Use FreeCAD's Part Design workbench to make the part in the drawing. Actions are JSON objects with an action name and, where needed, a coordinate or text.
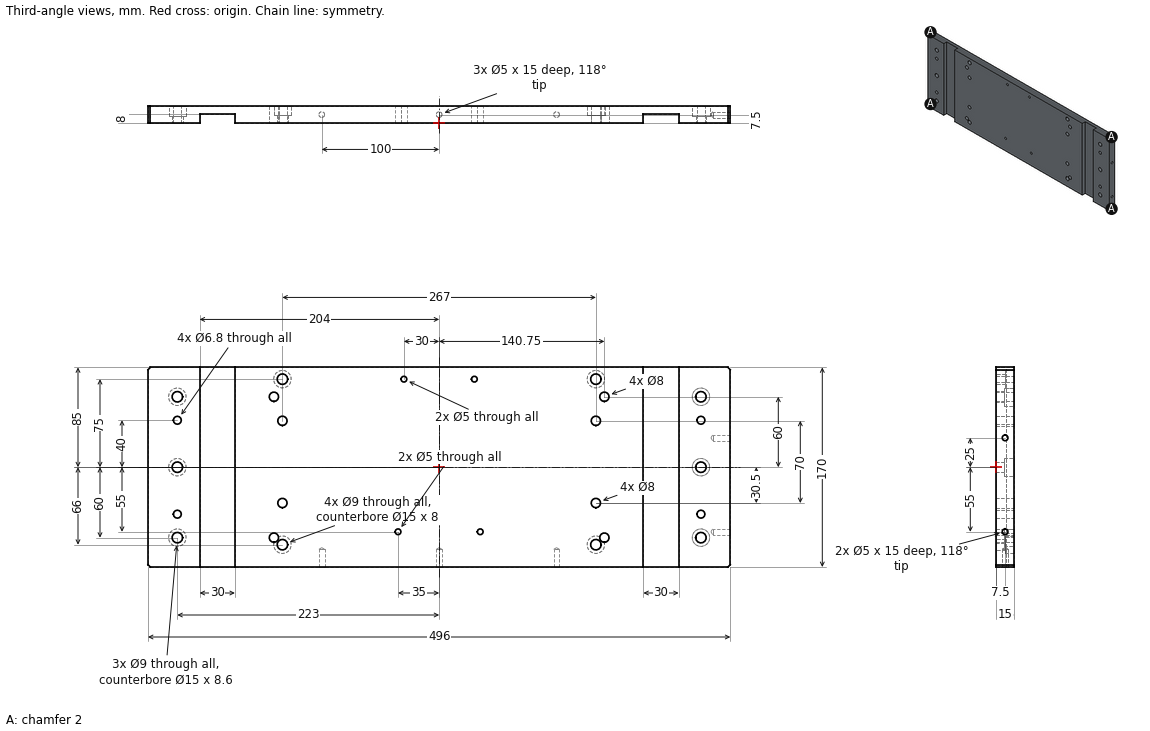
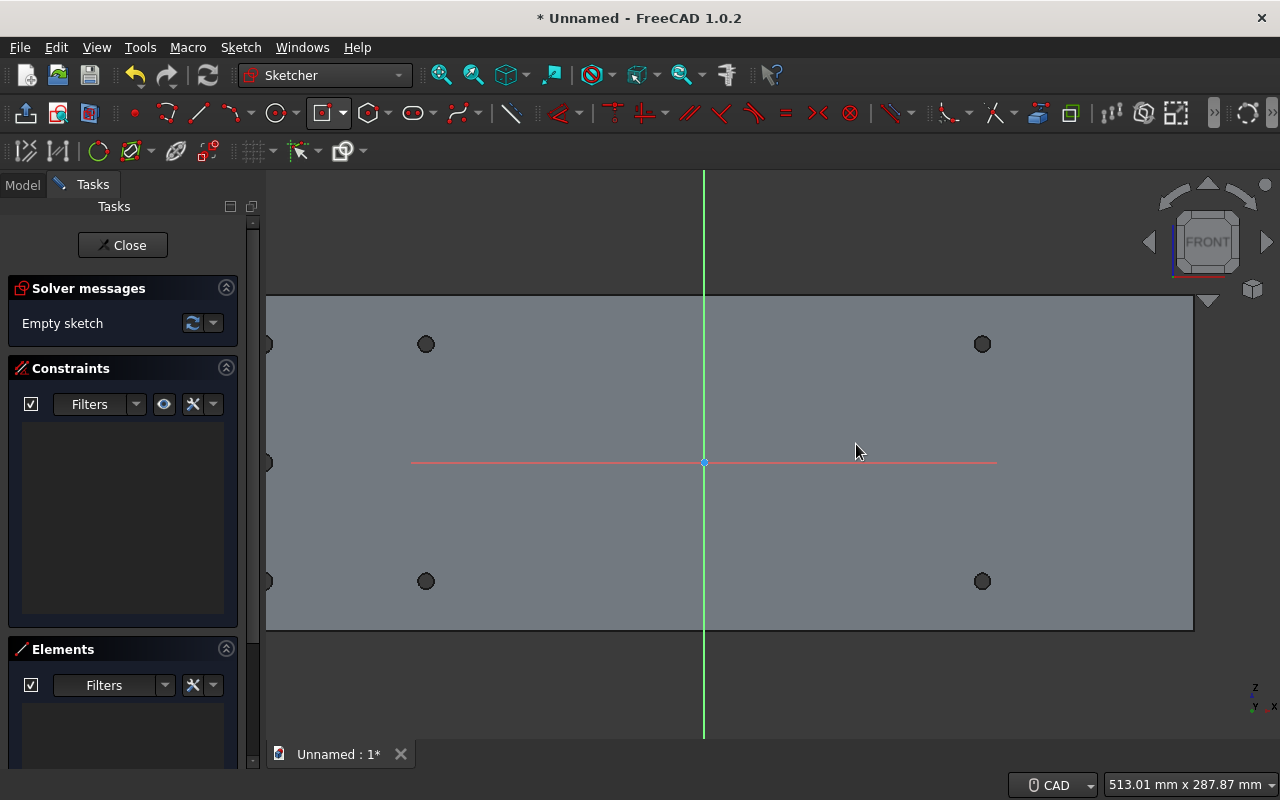
{"action": "left_click", "coordinate": [276, 114]}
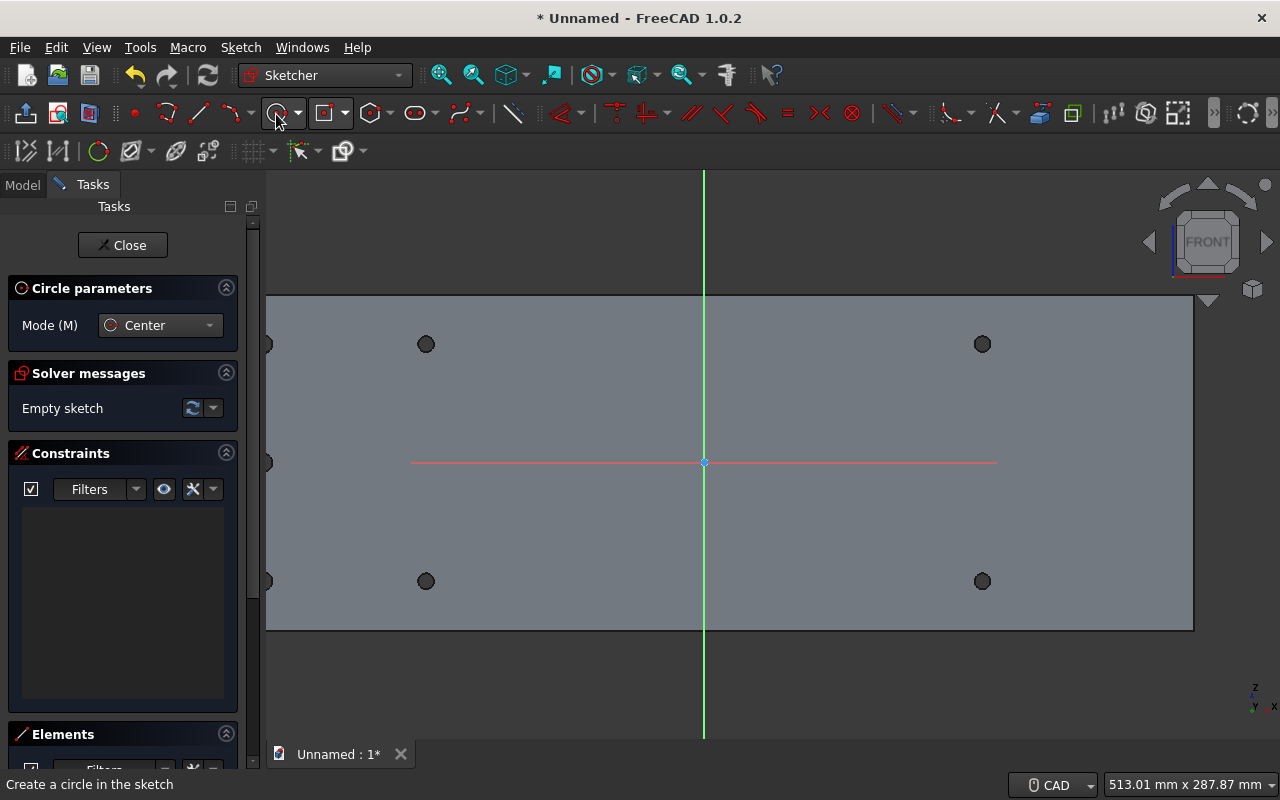
{"action": "scroll", "coordinate": [968, 523], "scroll_direction": "up", "scroll_amount": 6}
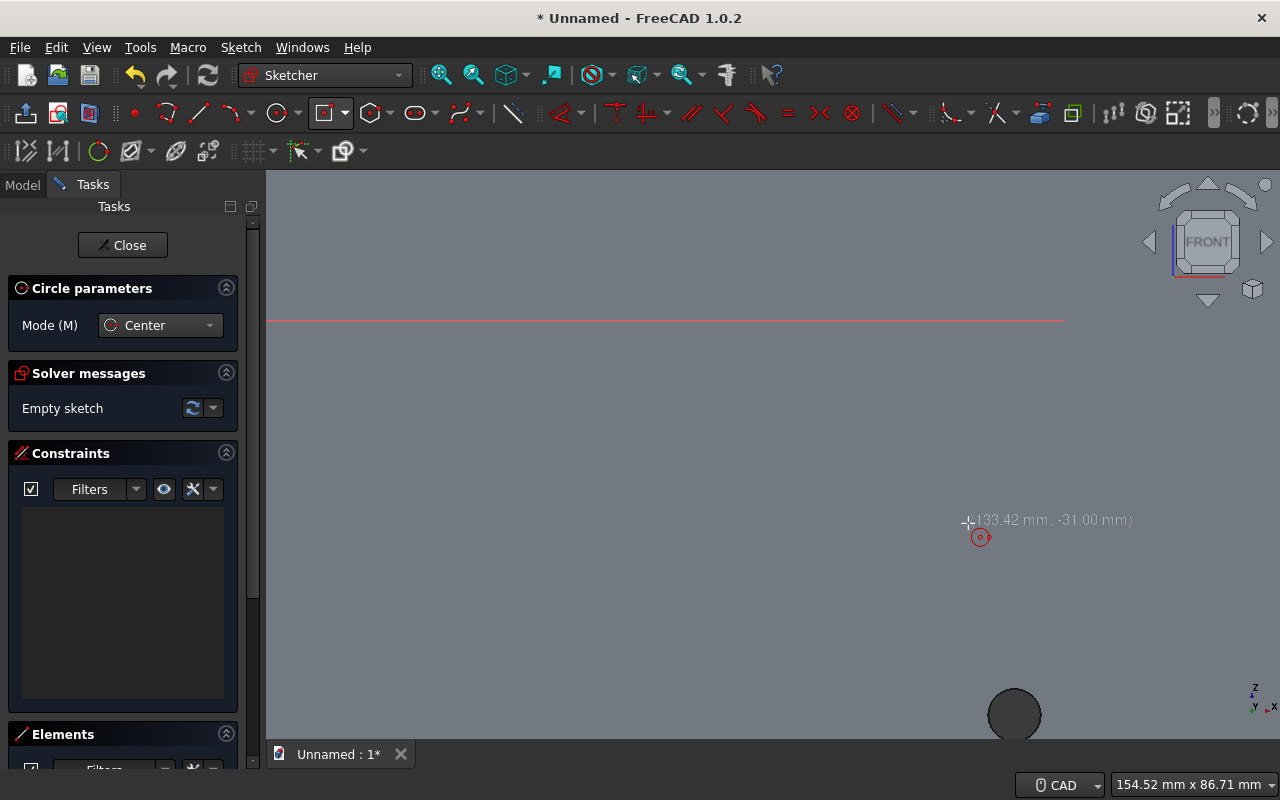
{"action": "left_click", "coordinate": [967, 522]}
{"action": "mouse_move", "coordinate": [985, 503]}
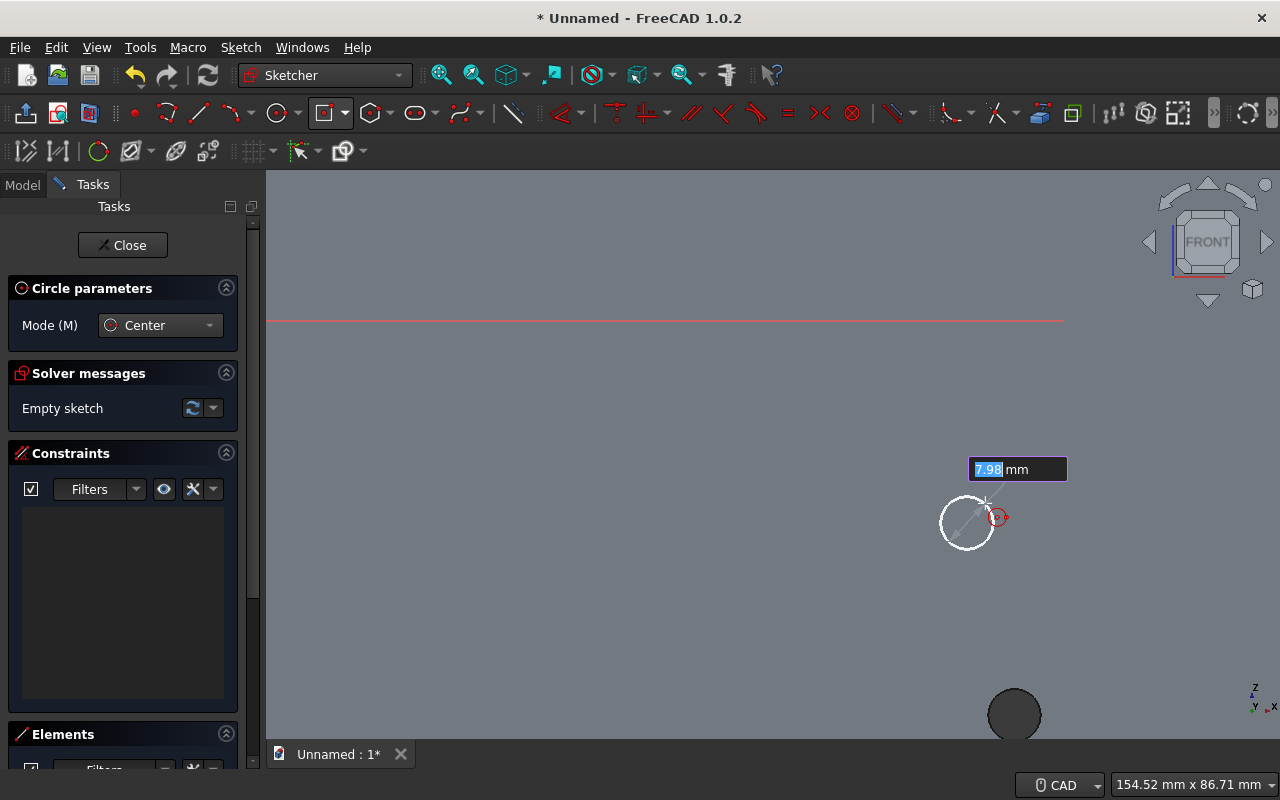
{"action": "type", "text": "8"}
{"action": "key", "text": "Return"}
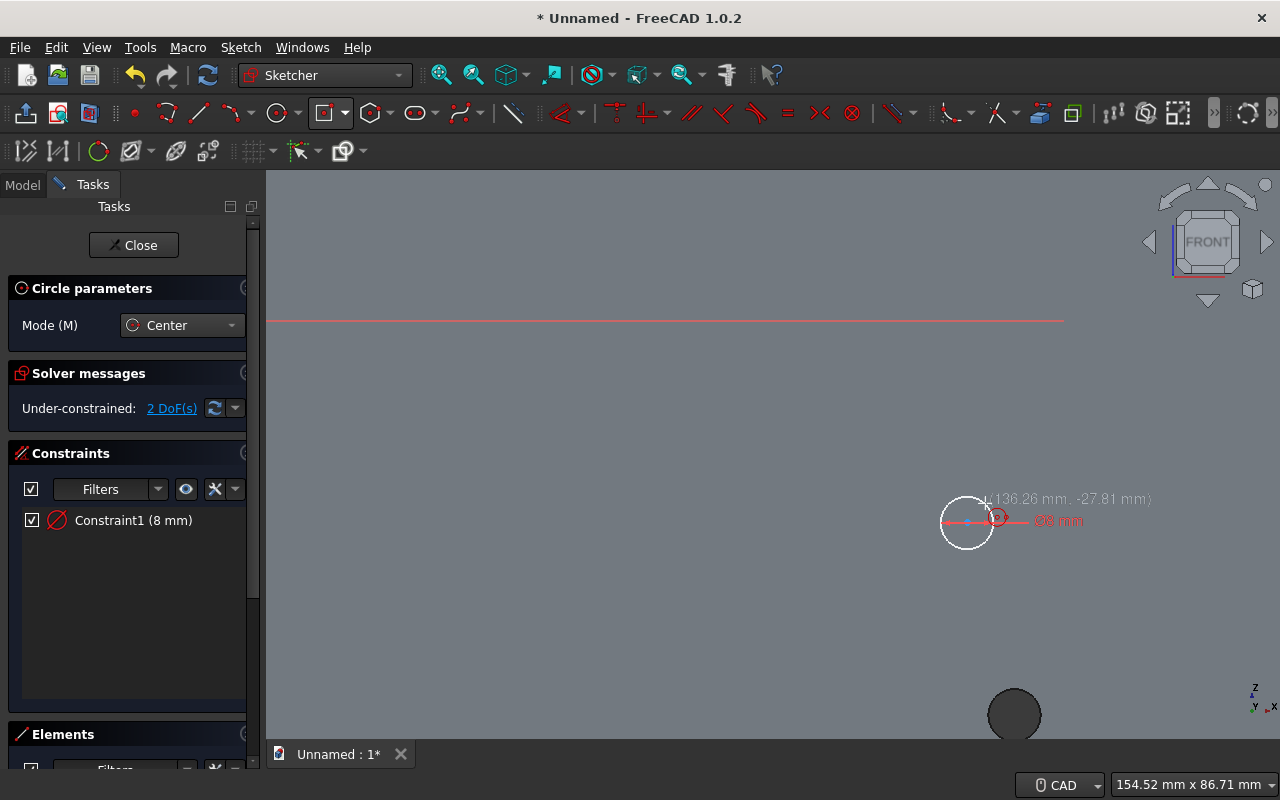
{"action": "scroll", "coordinate": [969, 525], "scroll_direction": "down", "scroll_amount": 6}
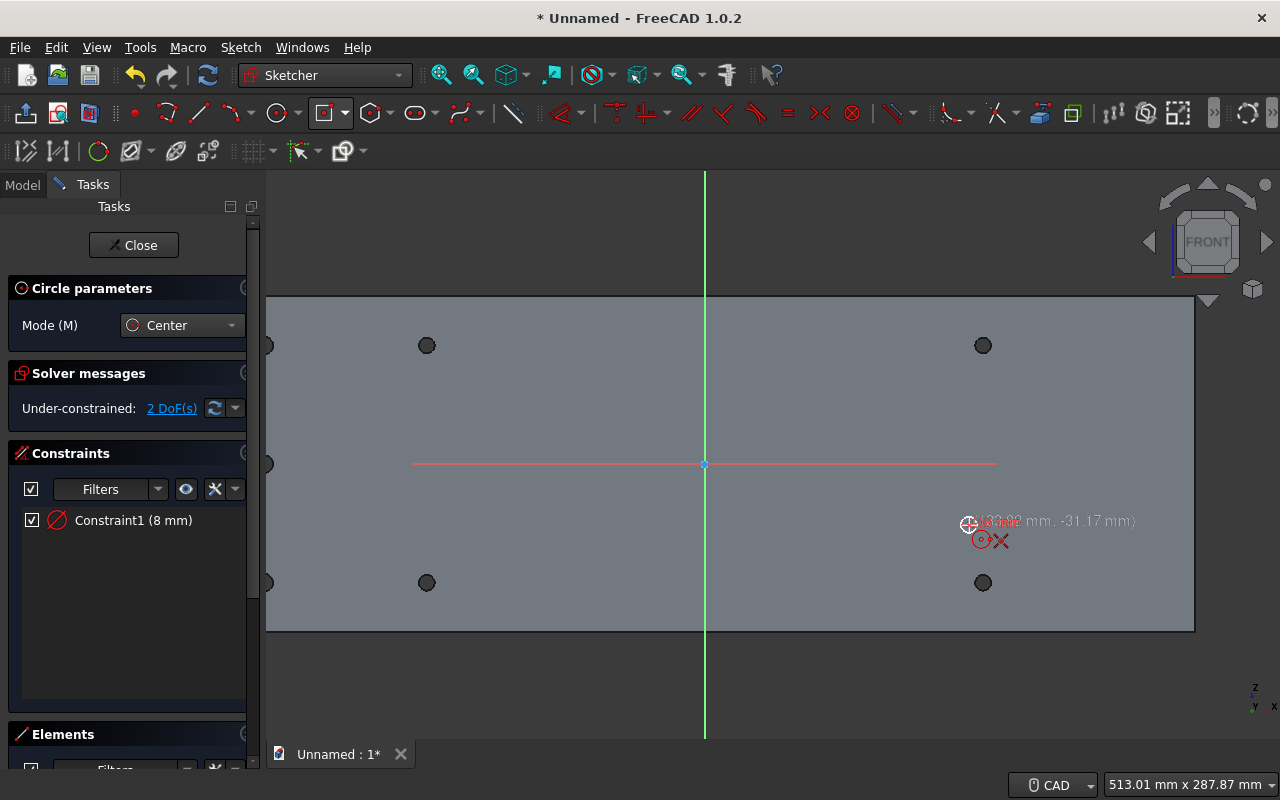
{"action": "scroll", "coordinate": [969, 386], "scroll_direction": "up", "scroll_amount": 6}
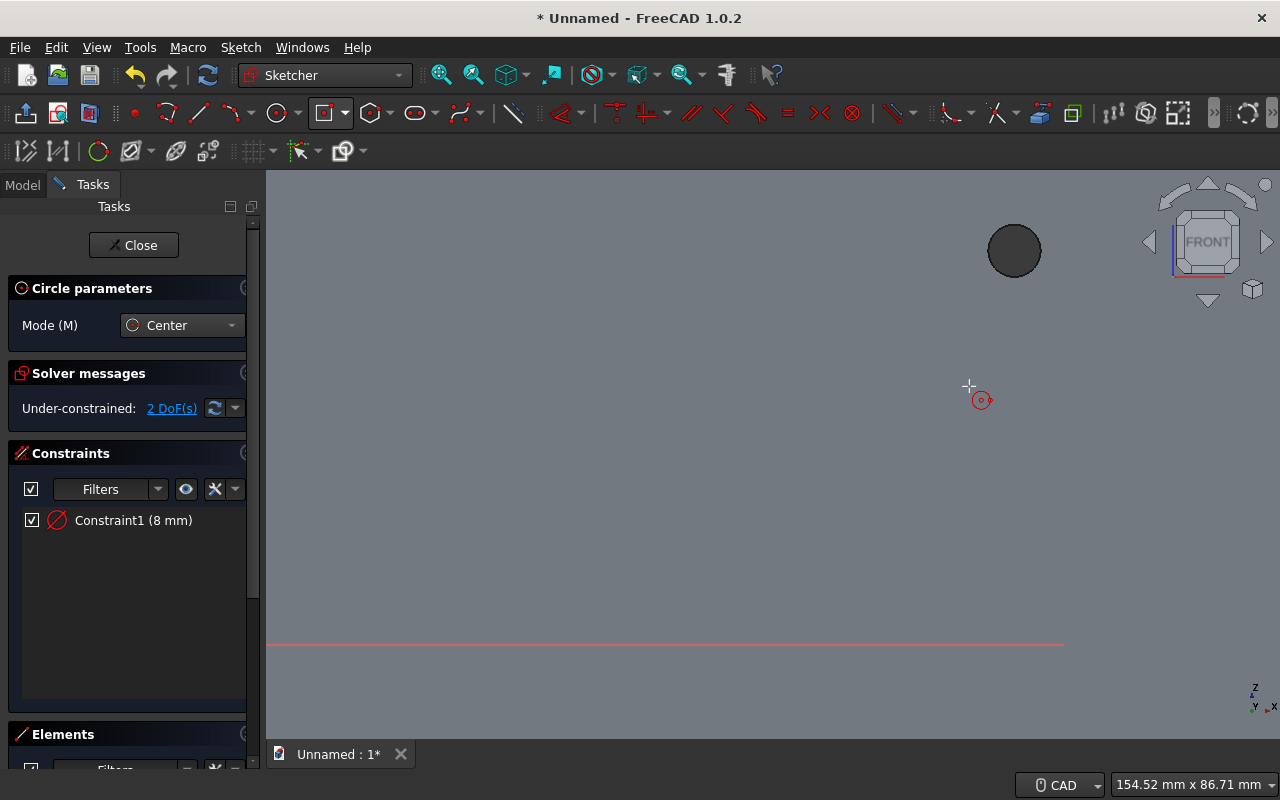
{"action": "left_click", "coordinate": [967, 385]}
{"action": "mouse_move", "coordinate": [985, 367]}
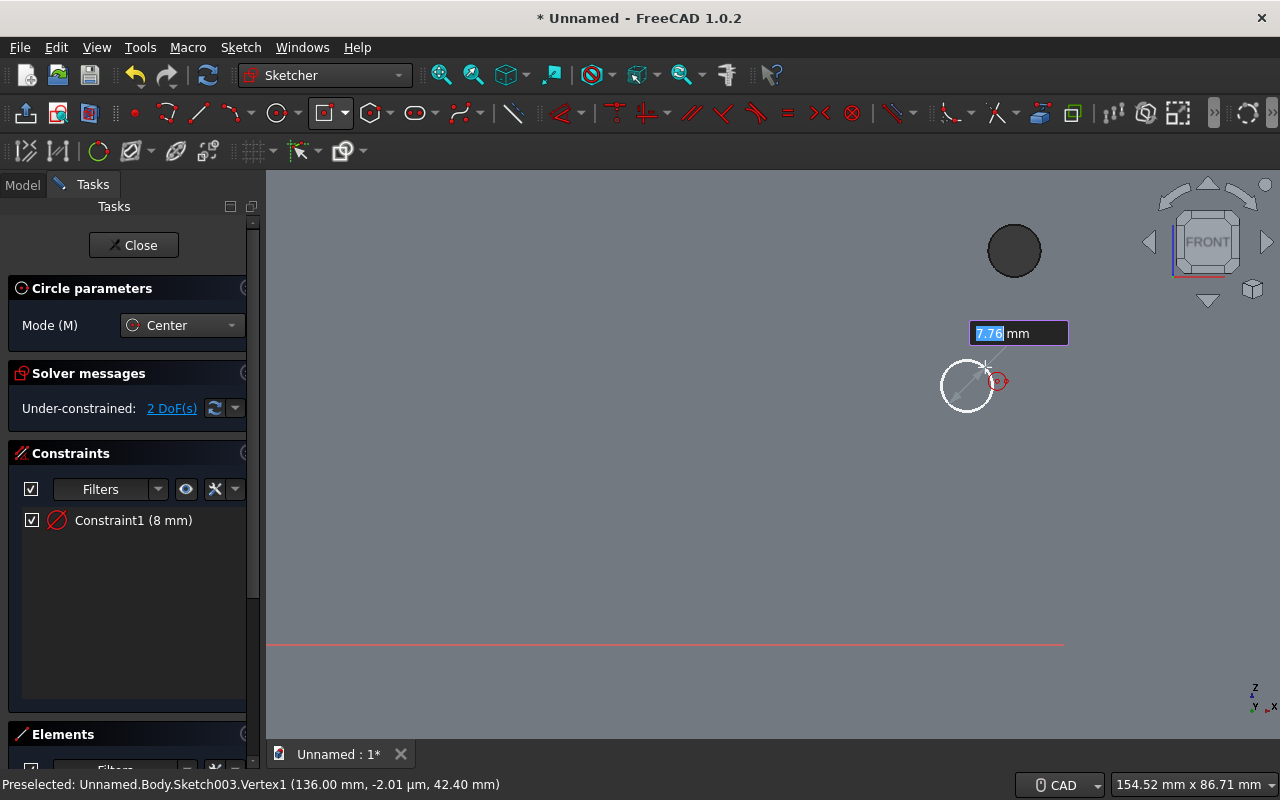
{"action": "type", "text": "8"}
{"action": "key", "text": "Return"}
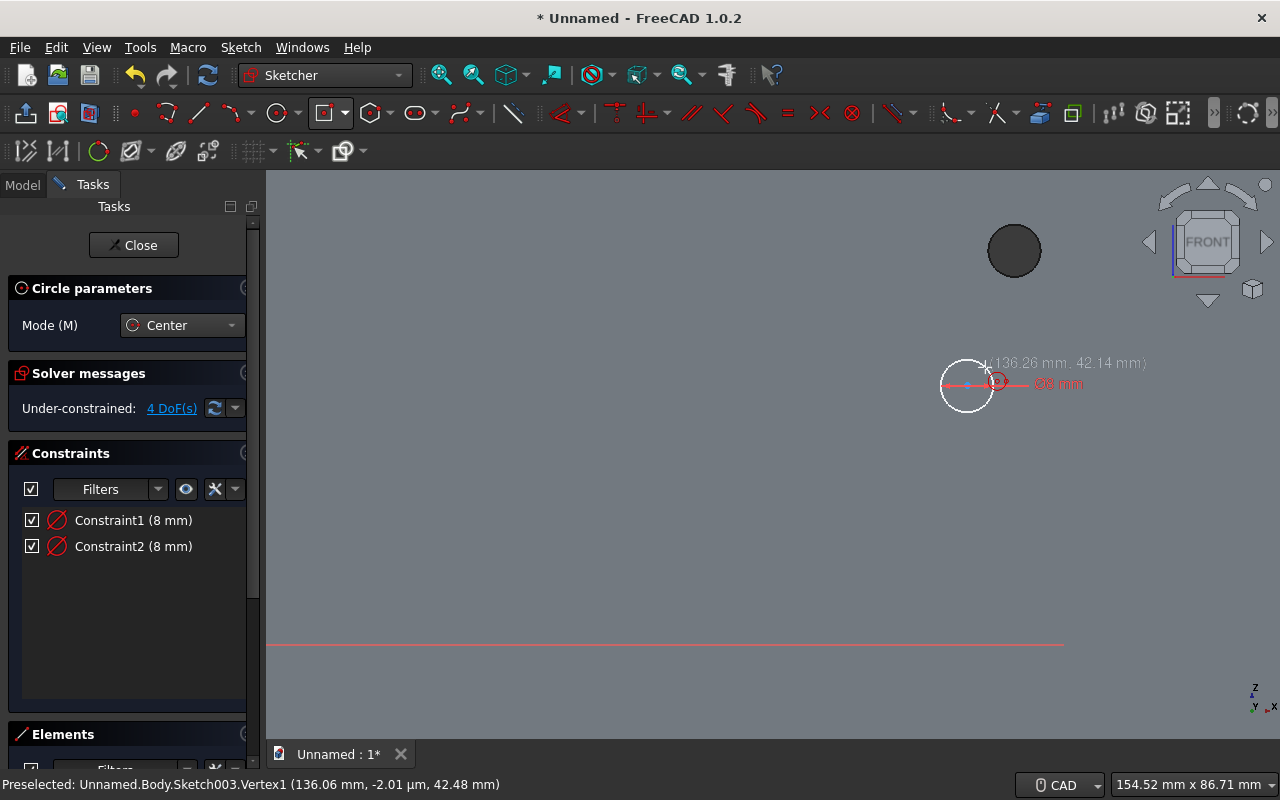
{"action": "scroll", "coordinate": [969, 385], "scroll_direction": "down", "scroll_amount": 6}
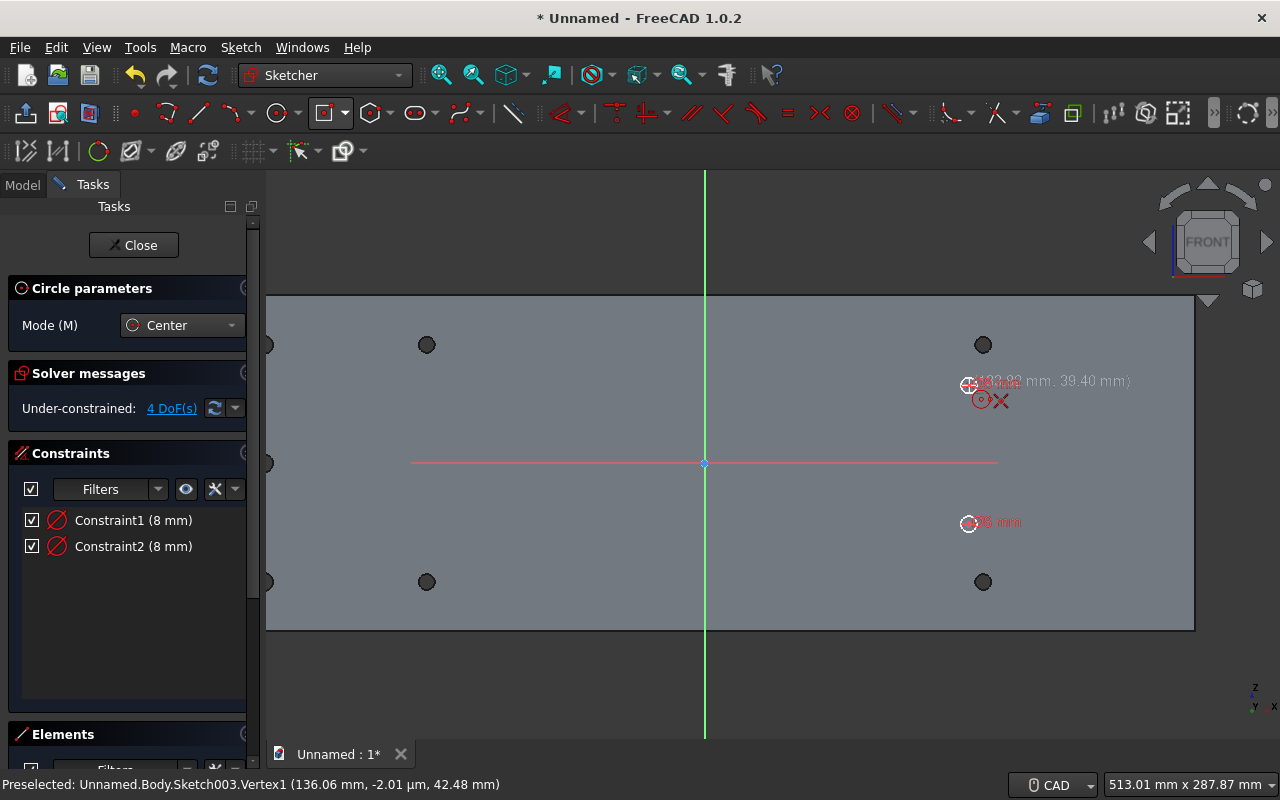
{"action": "scroll", "coordinate": [441, 385], "scroll_direction": "up", "scroll_amount": 6}